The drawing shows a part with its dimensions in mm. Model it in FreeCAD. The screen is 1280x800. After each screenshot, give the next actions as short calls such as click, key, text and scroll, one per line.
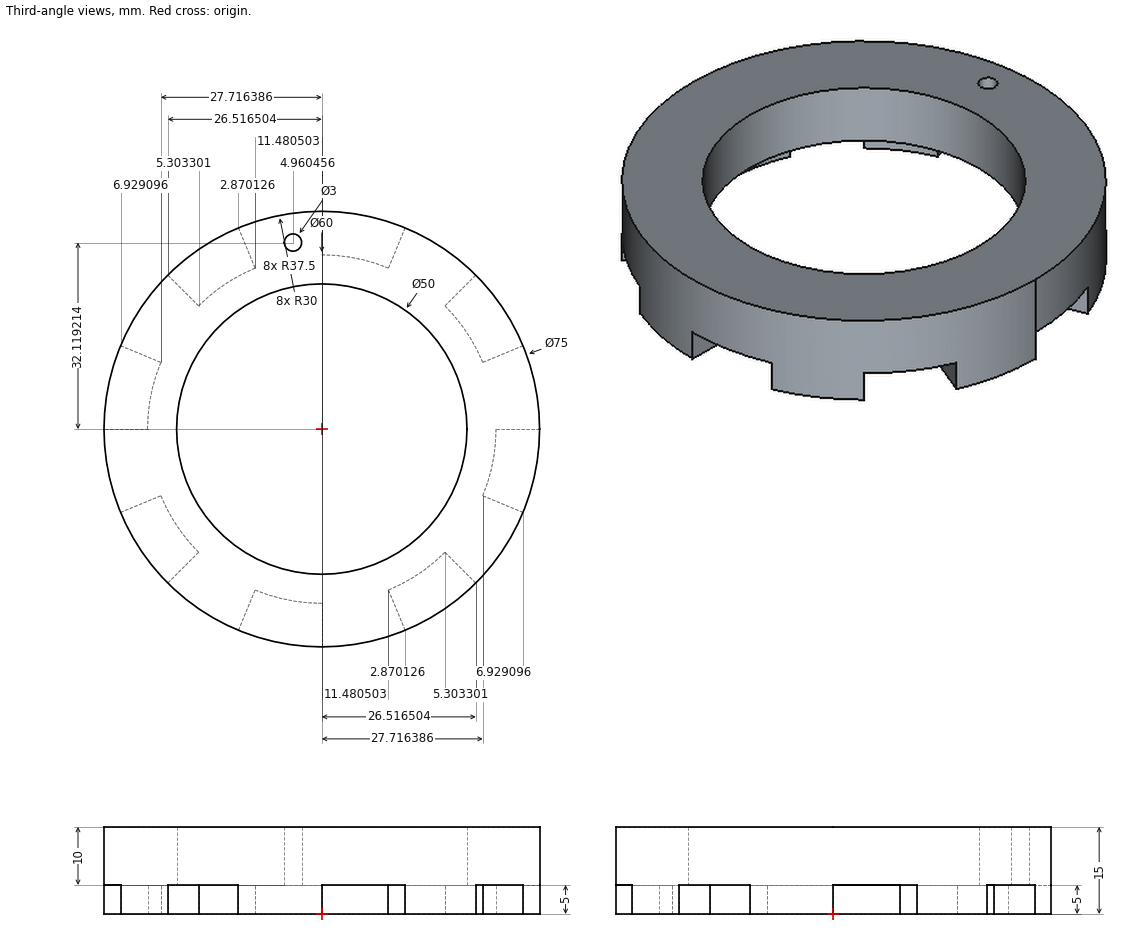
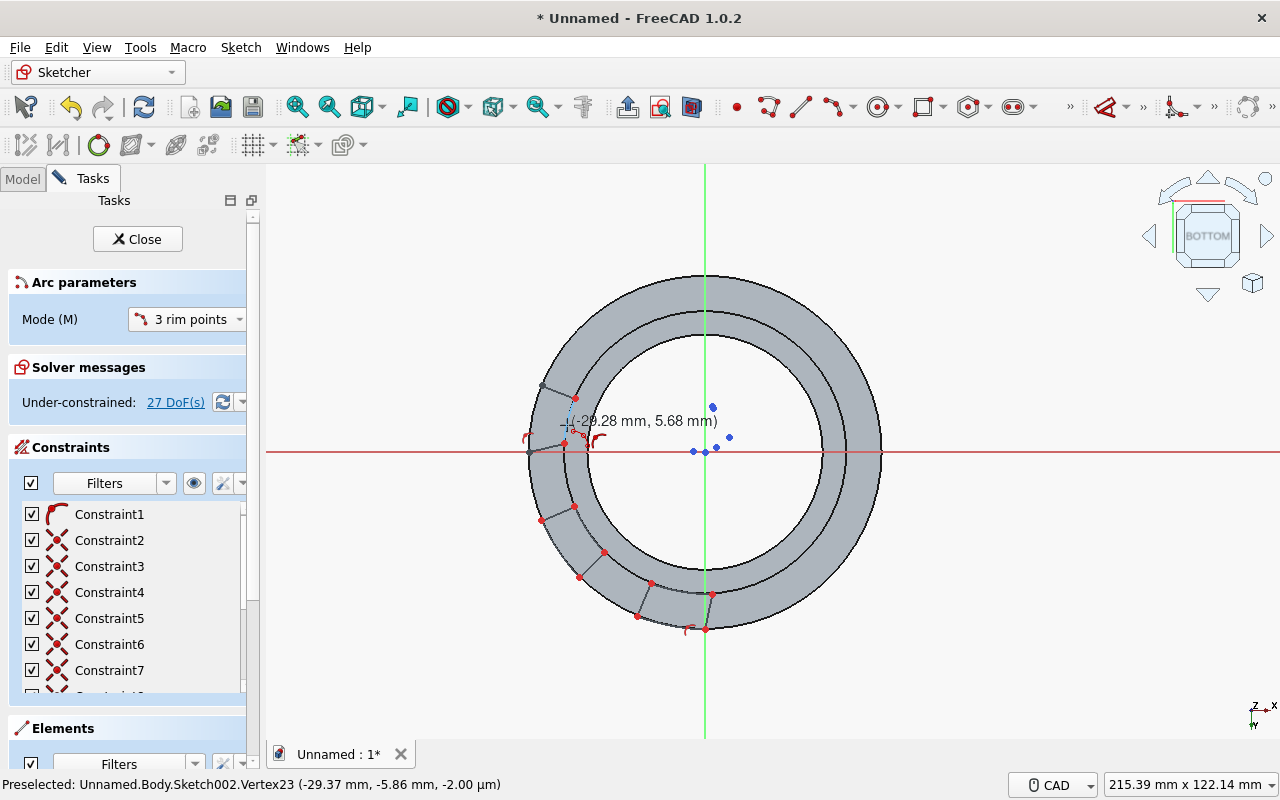
click(542, 386)
click(529, 452)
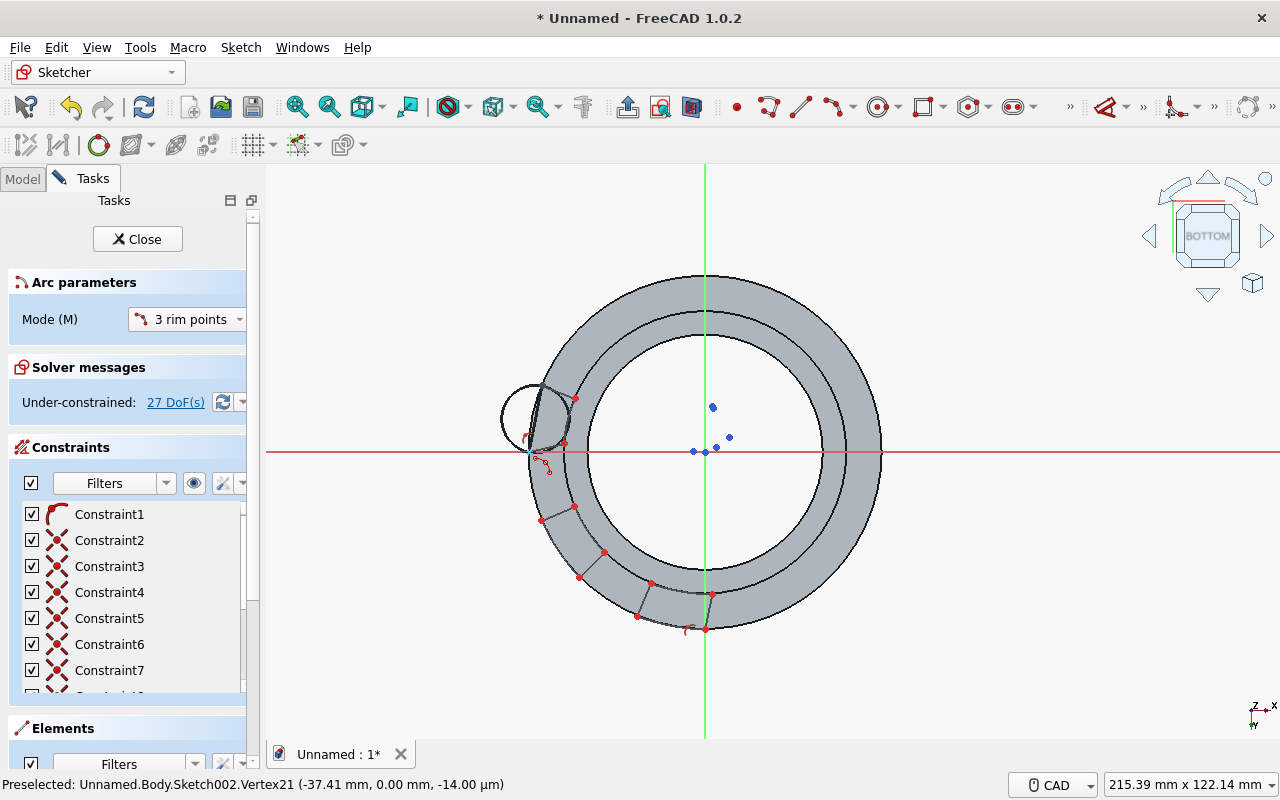
scroll(532, 418, up, 8)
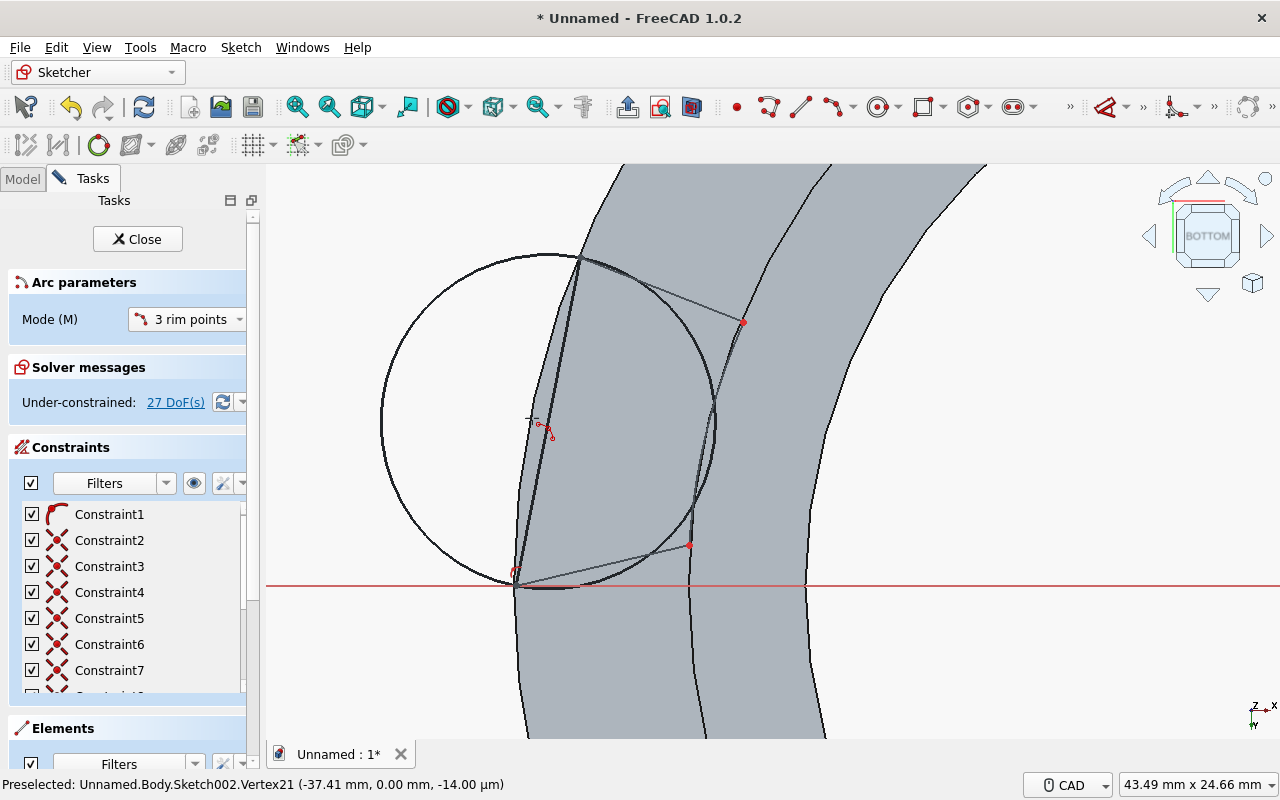
click(531, 415)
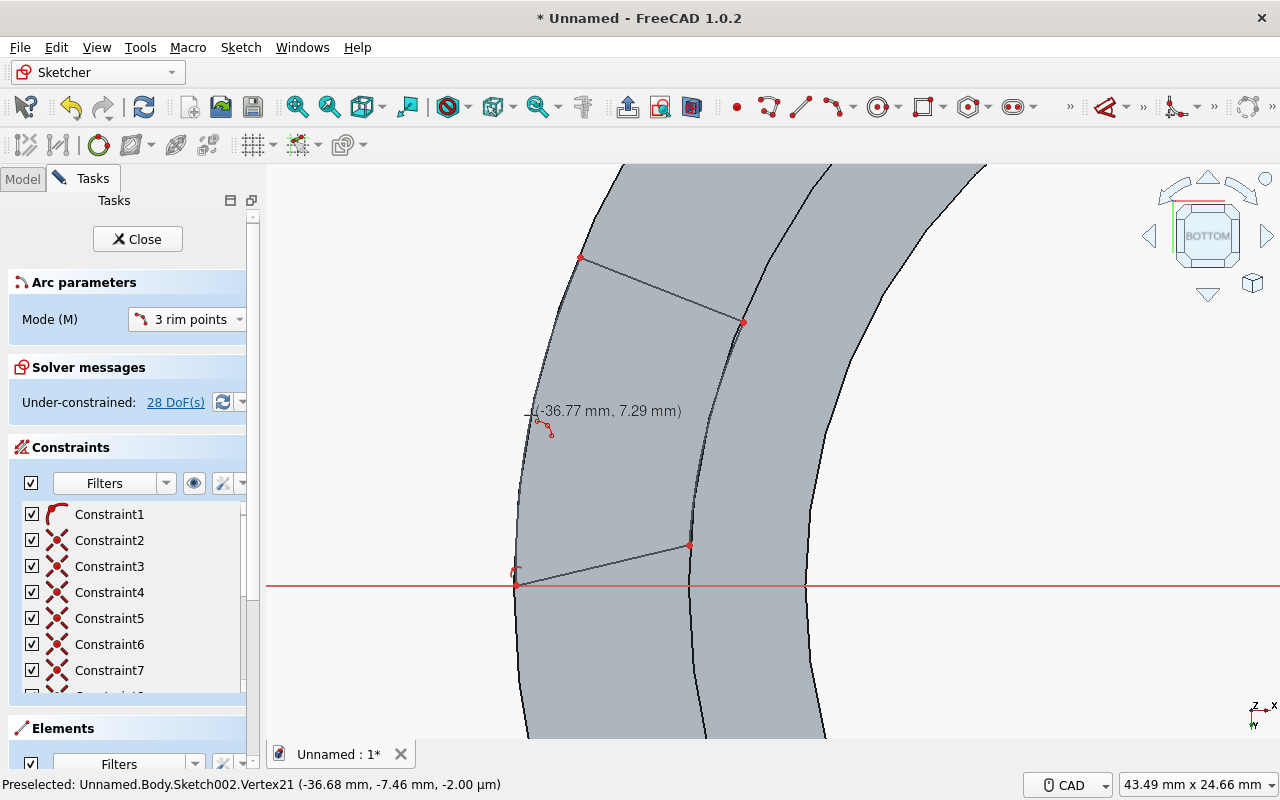
key(g)
key(l)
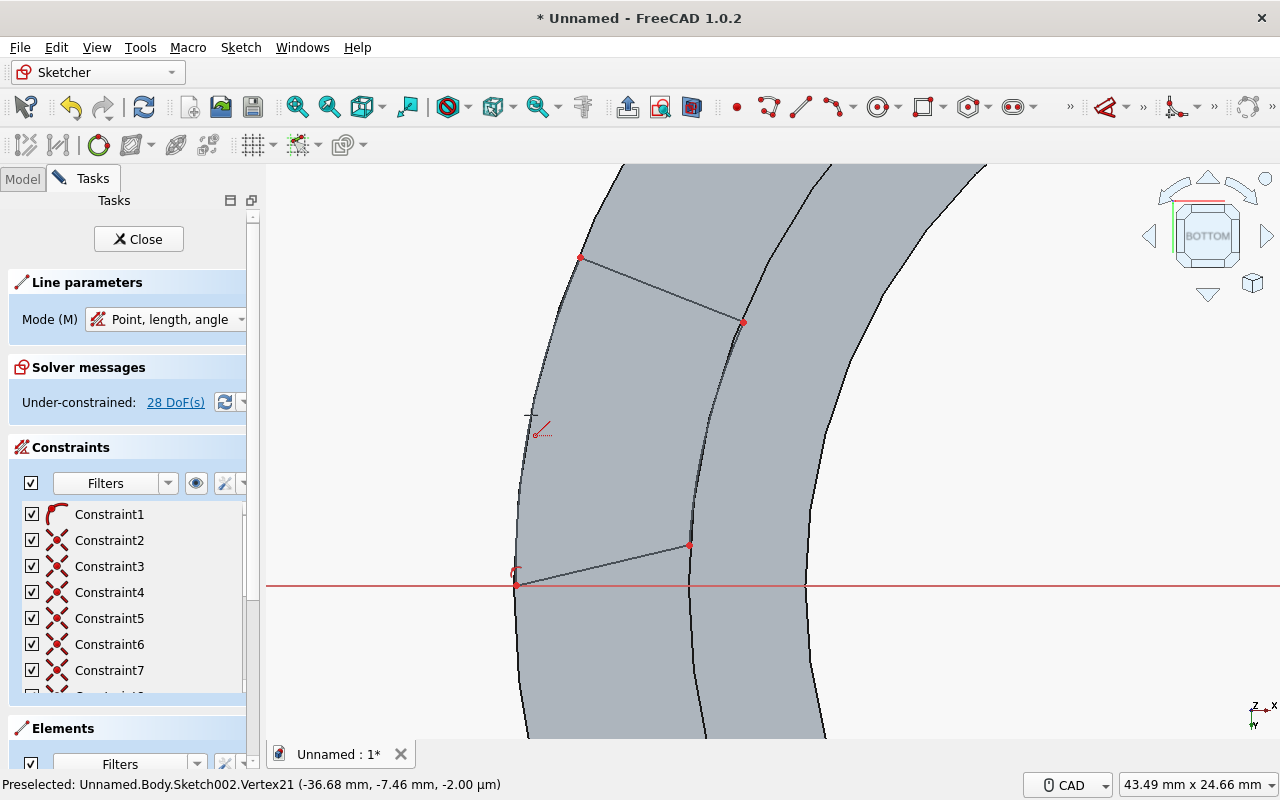
scroll(532, 417, down, 8)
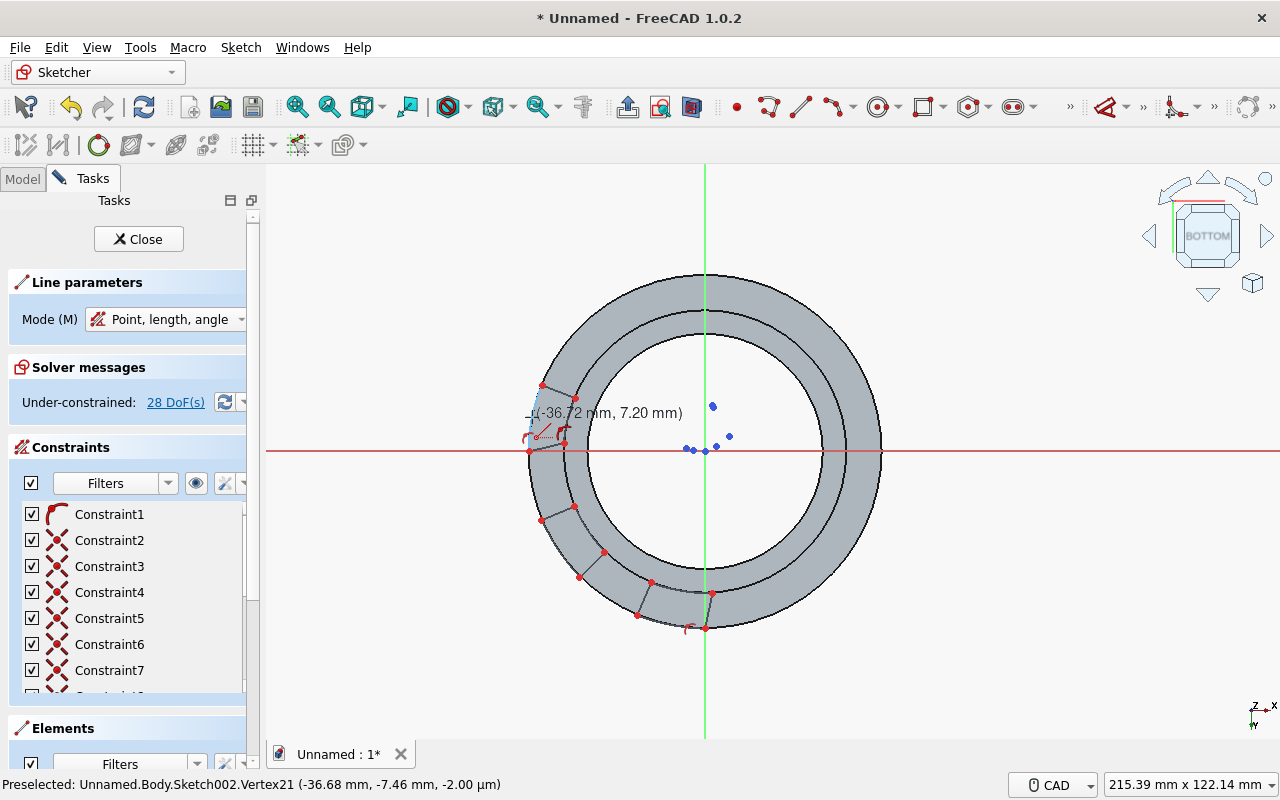
click(580, 327)
click(605, 352)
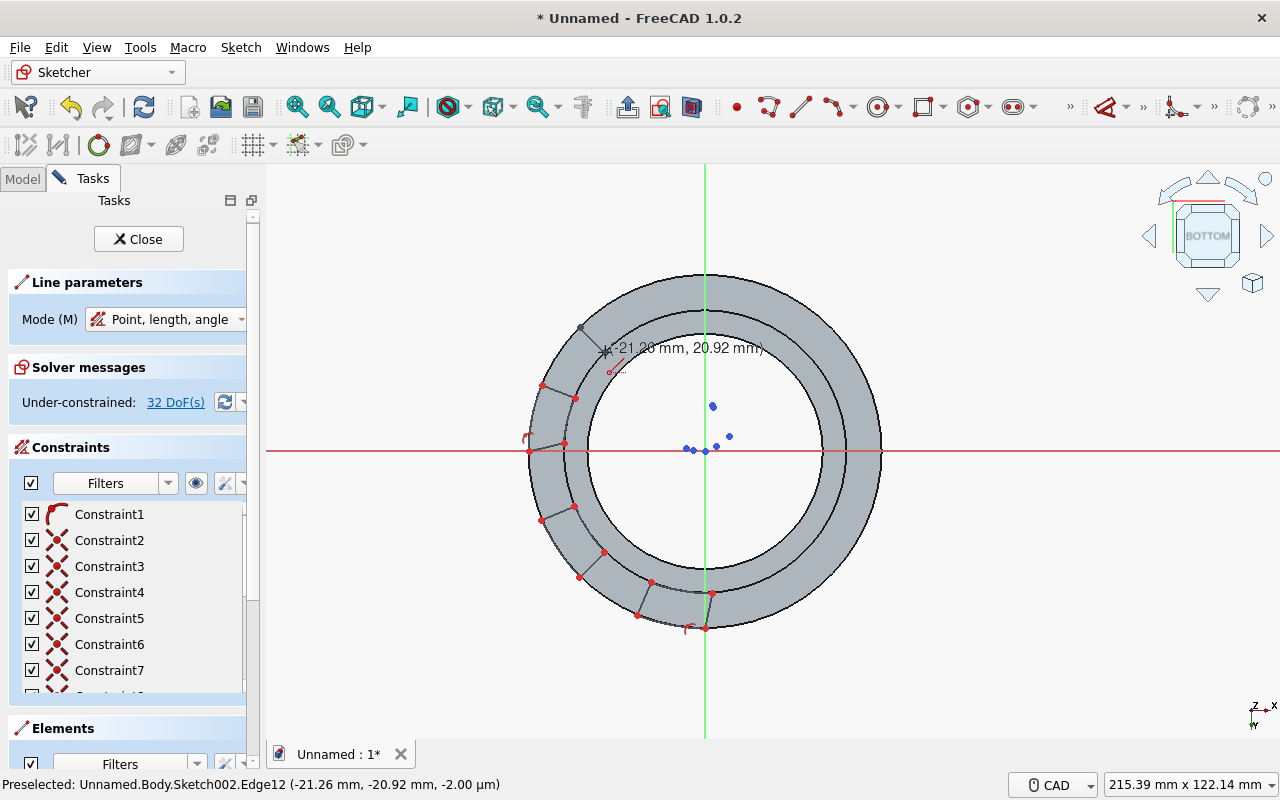
click(651, 321)
click(638, 288)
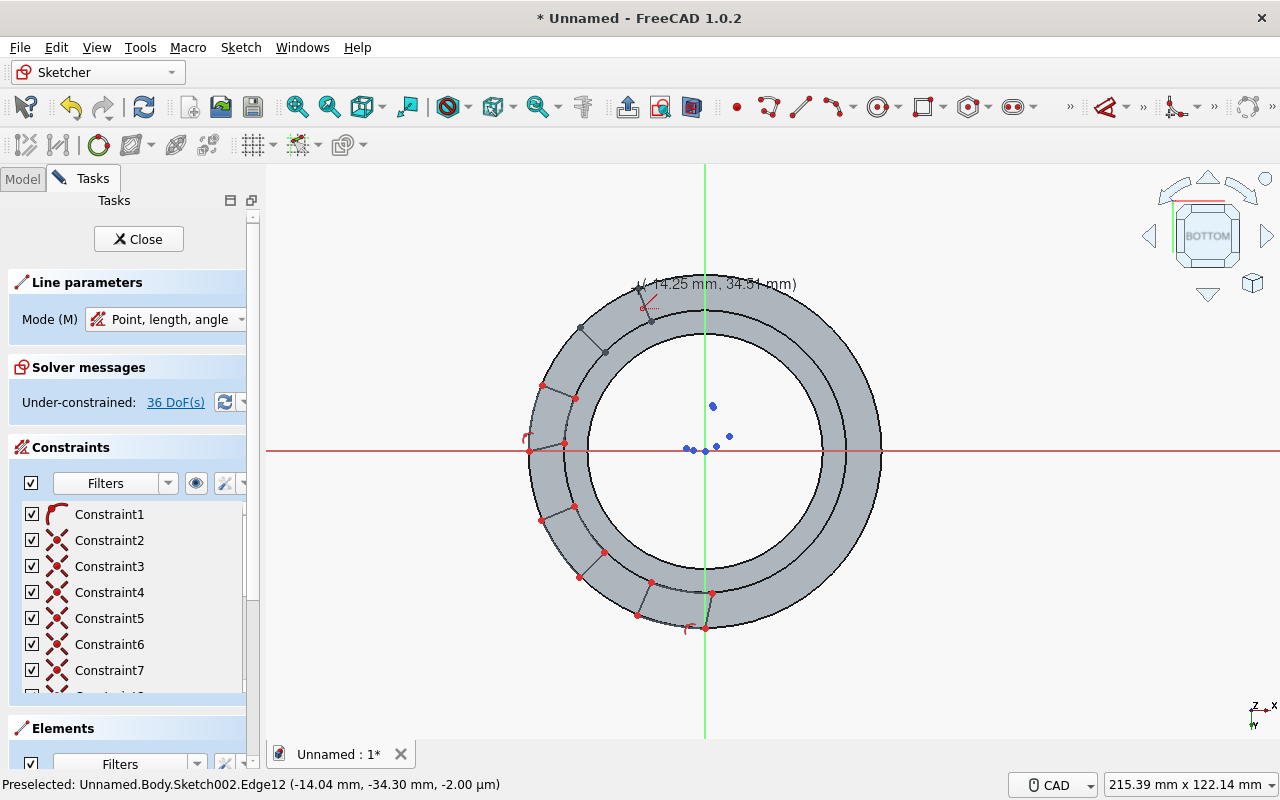
key(g)
key(3)
key(a)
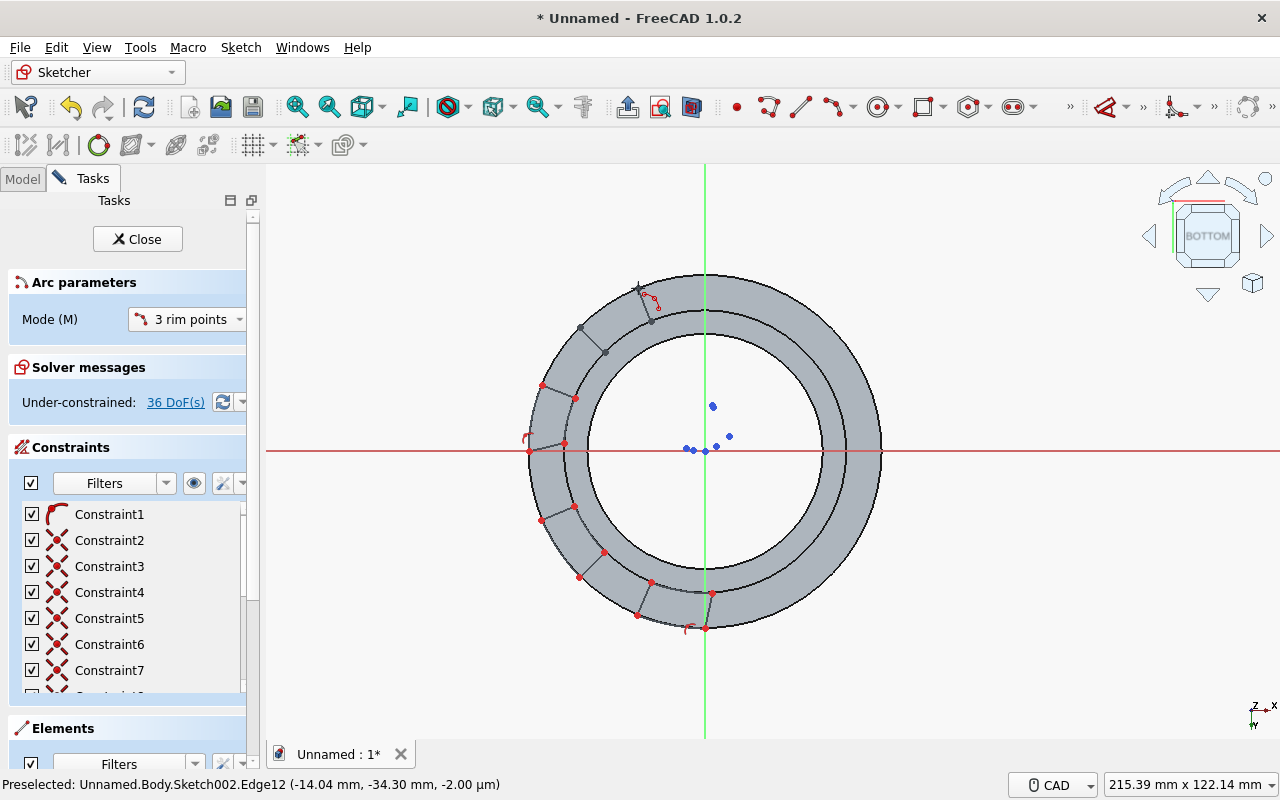
click(605, 353)
click(651, 322)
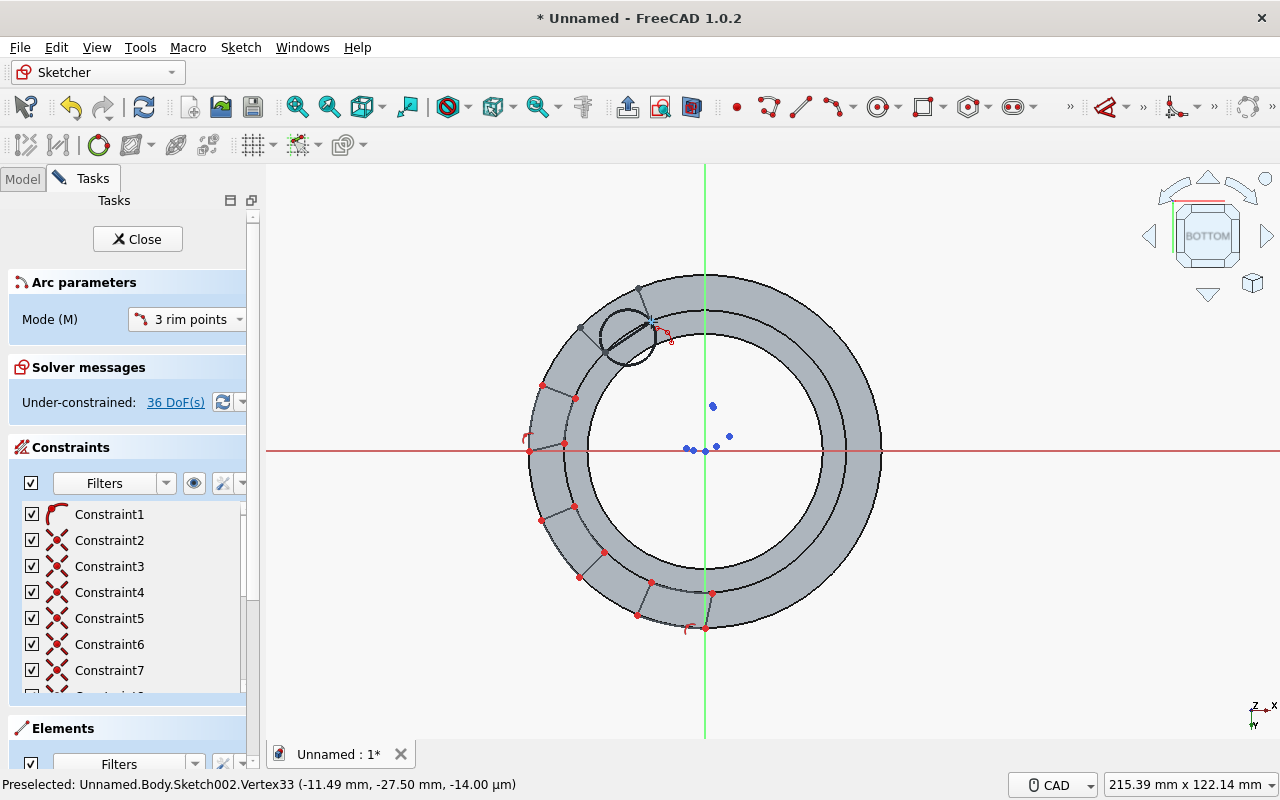
scroll(627, 334, up, 9)